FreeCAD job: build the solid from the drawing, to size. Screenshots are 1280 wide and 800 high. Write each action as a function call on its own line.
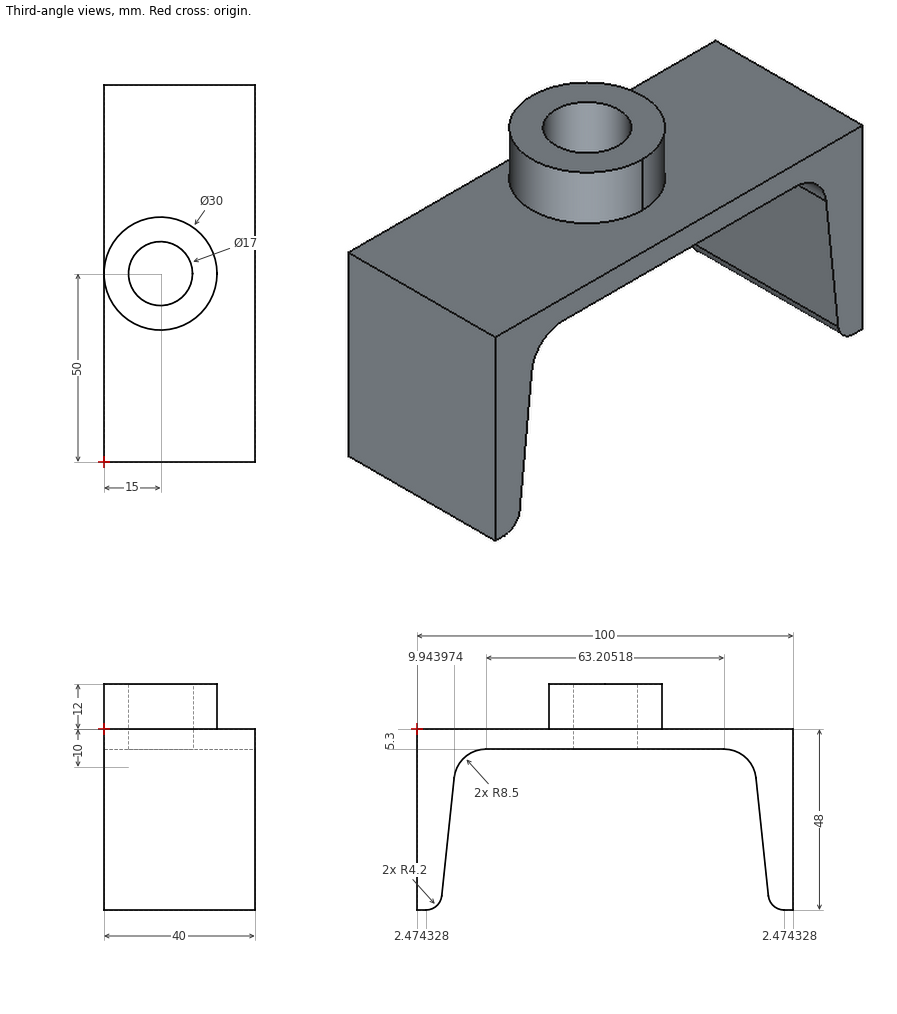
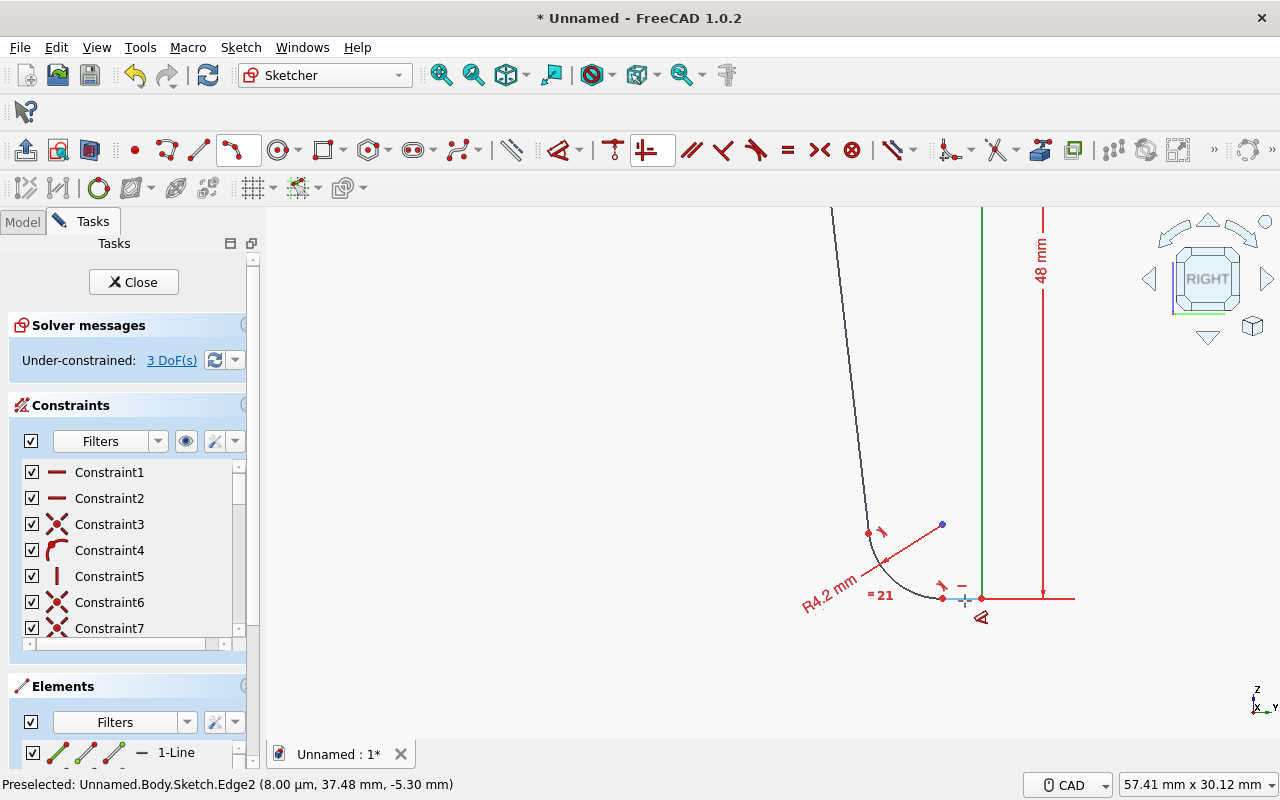
click(962, 599)
click(962, 633)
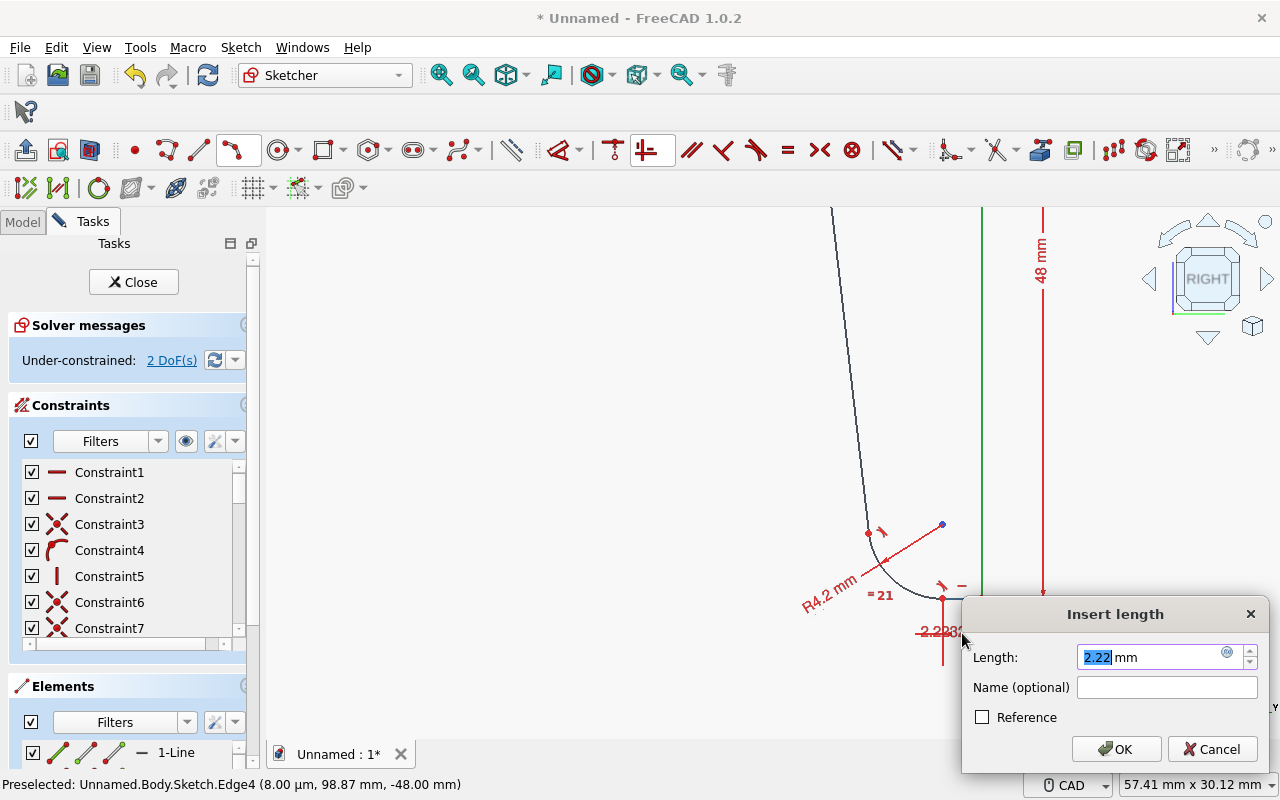
text(2.474328)
key(Return)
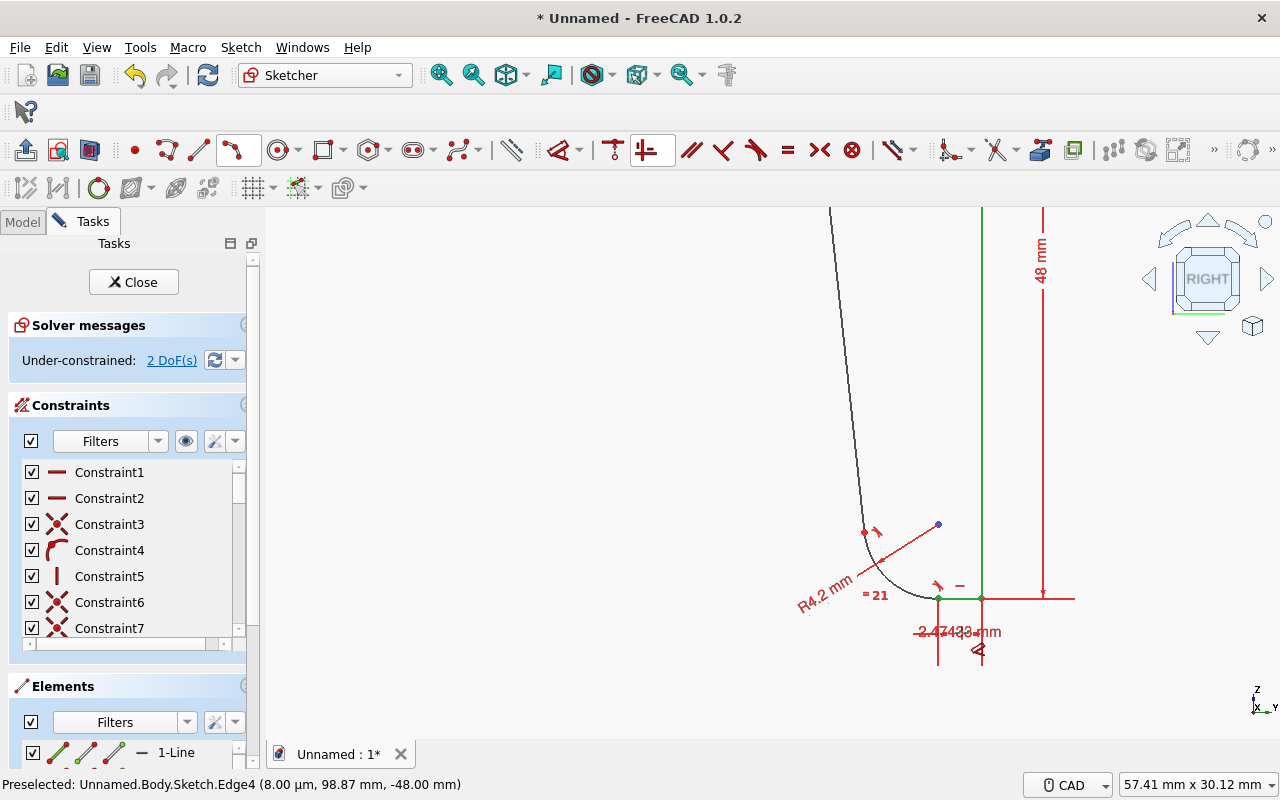
scroll(966, 601, down, 6)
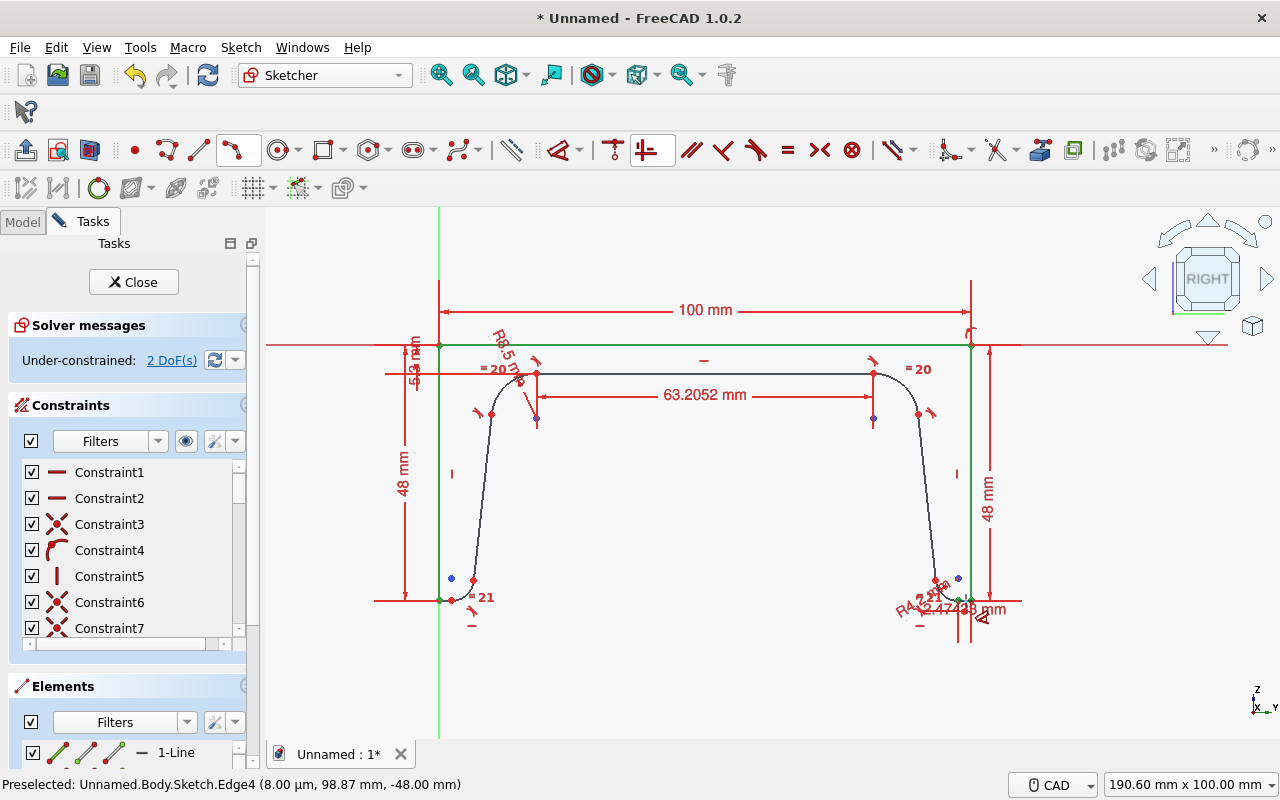
scroll(443, 601, up, 7)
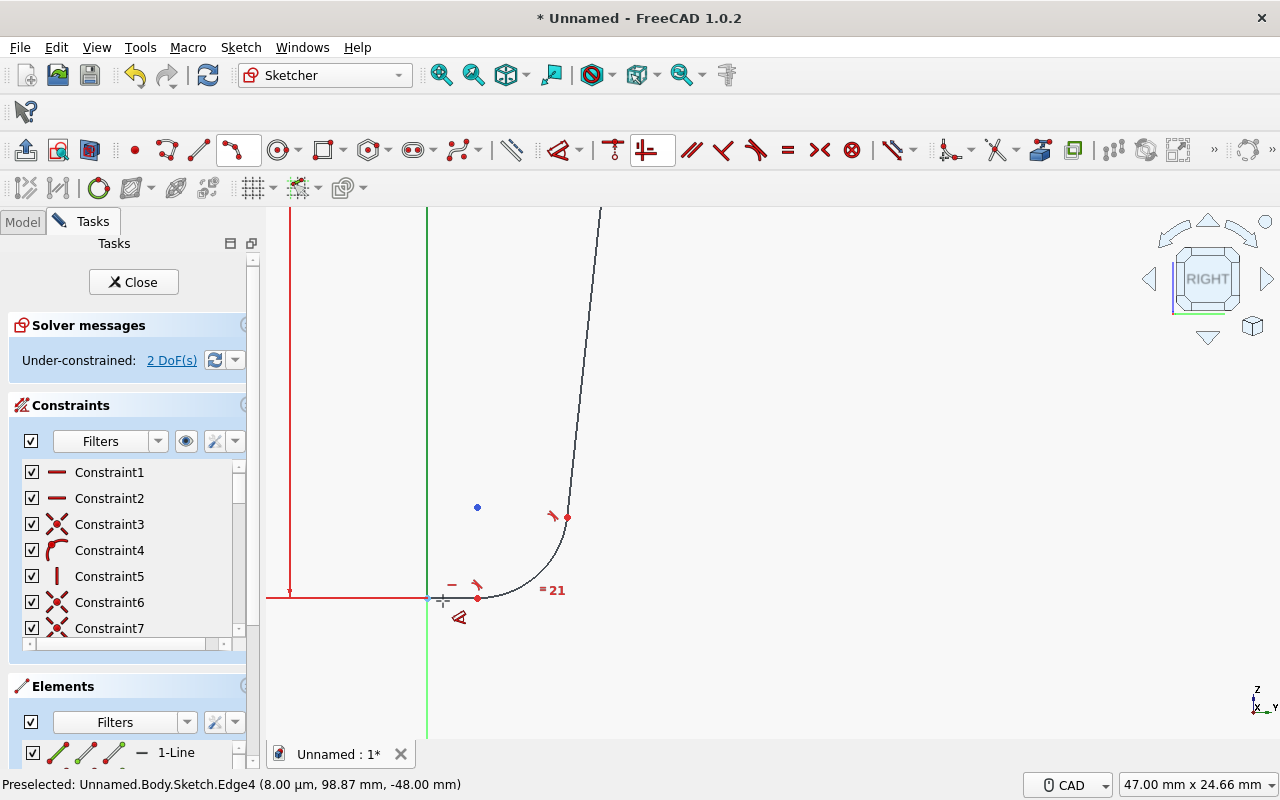
click(442, 598)
click(452, 632)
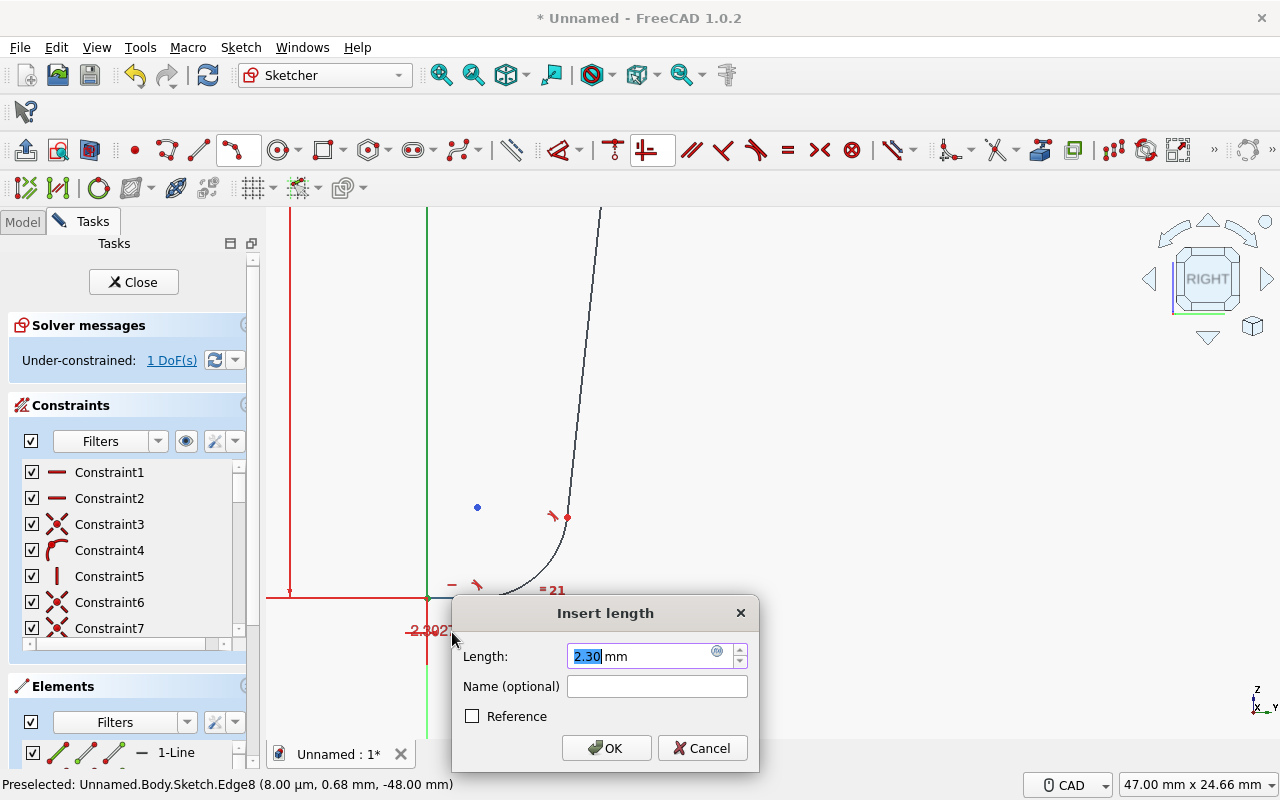
text(2.474328)
key(Return)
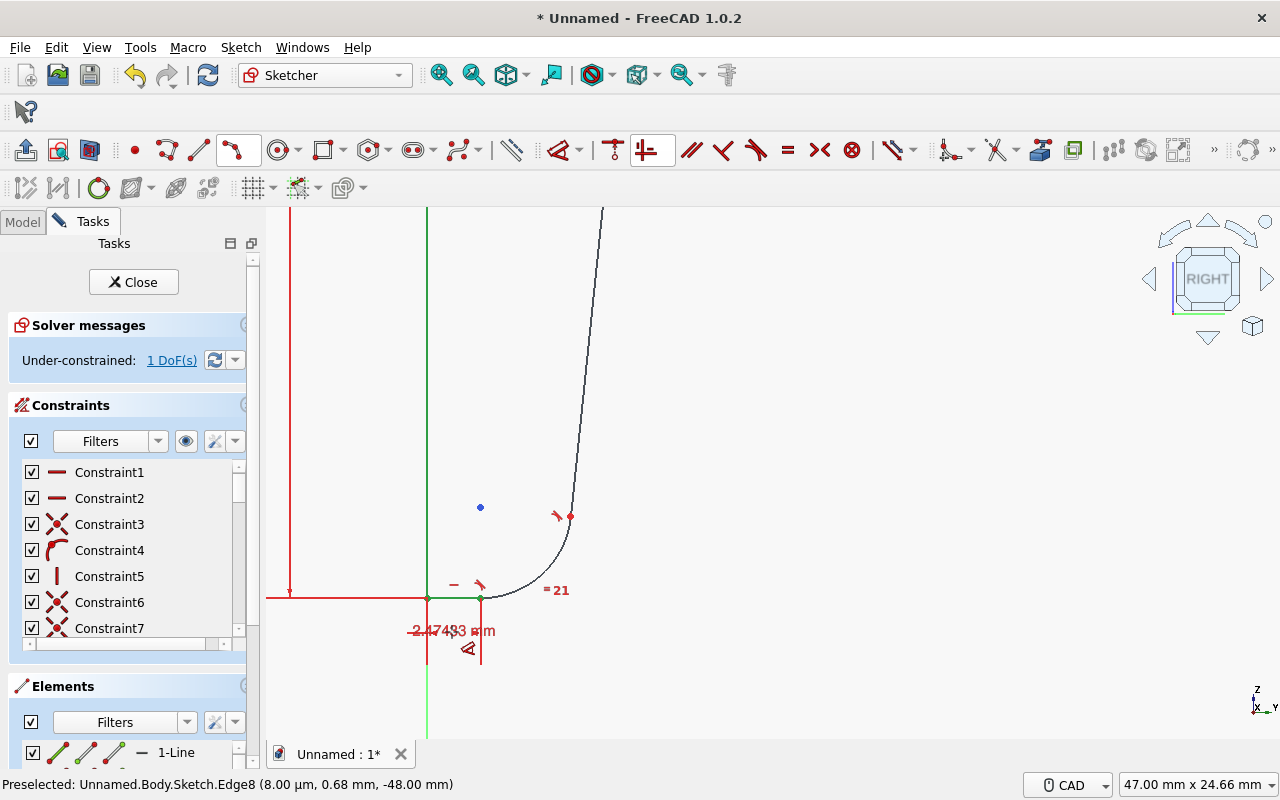
scroll(442, 602, down, 7)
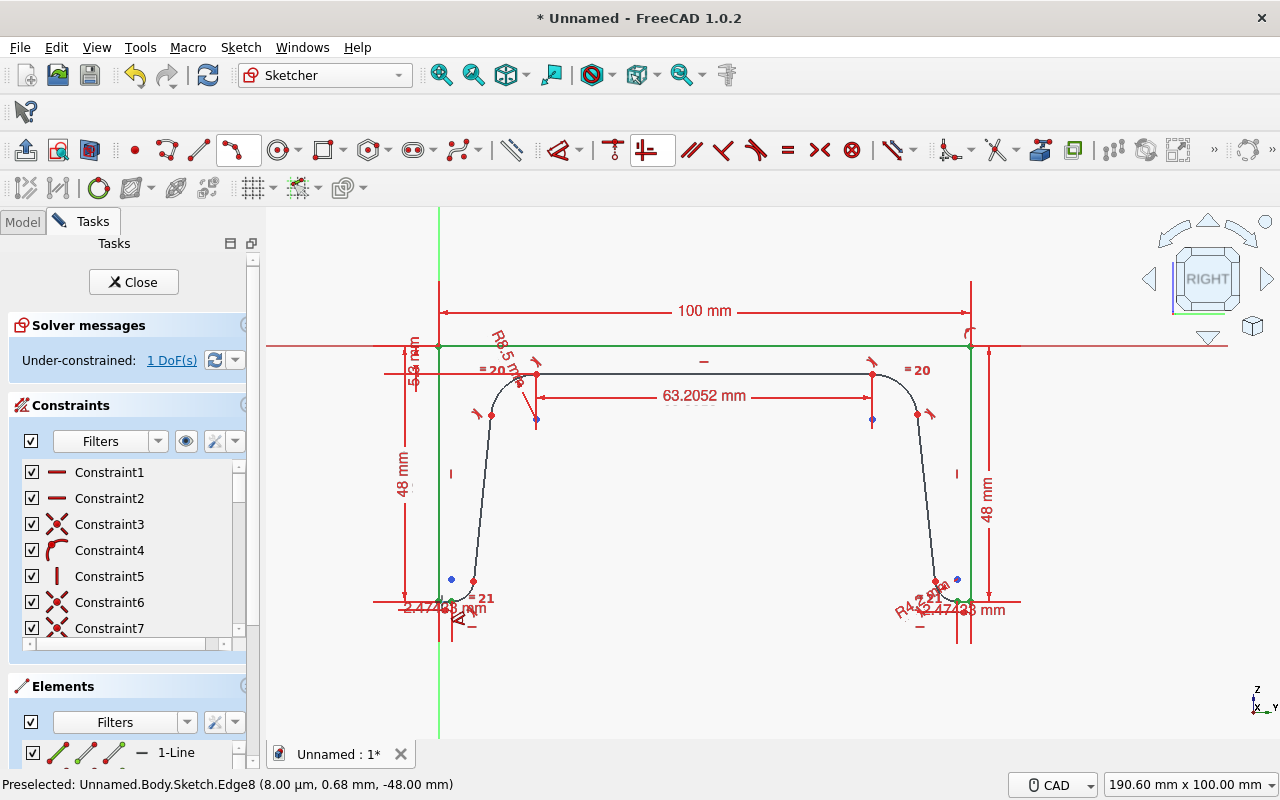
click(491, 415)
click(465, 312)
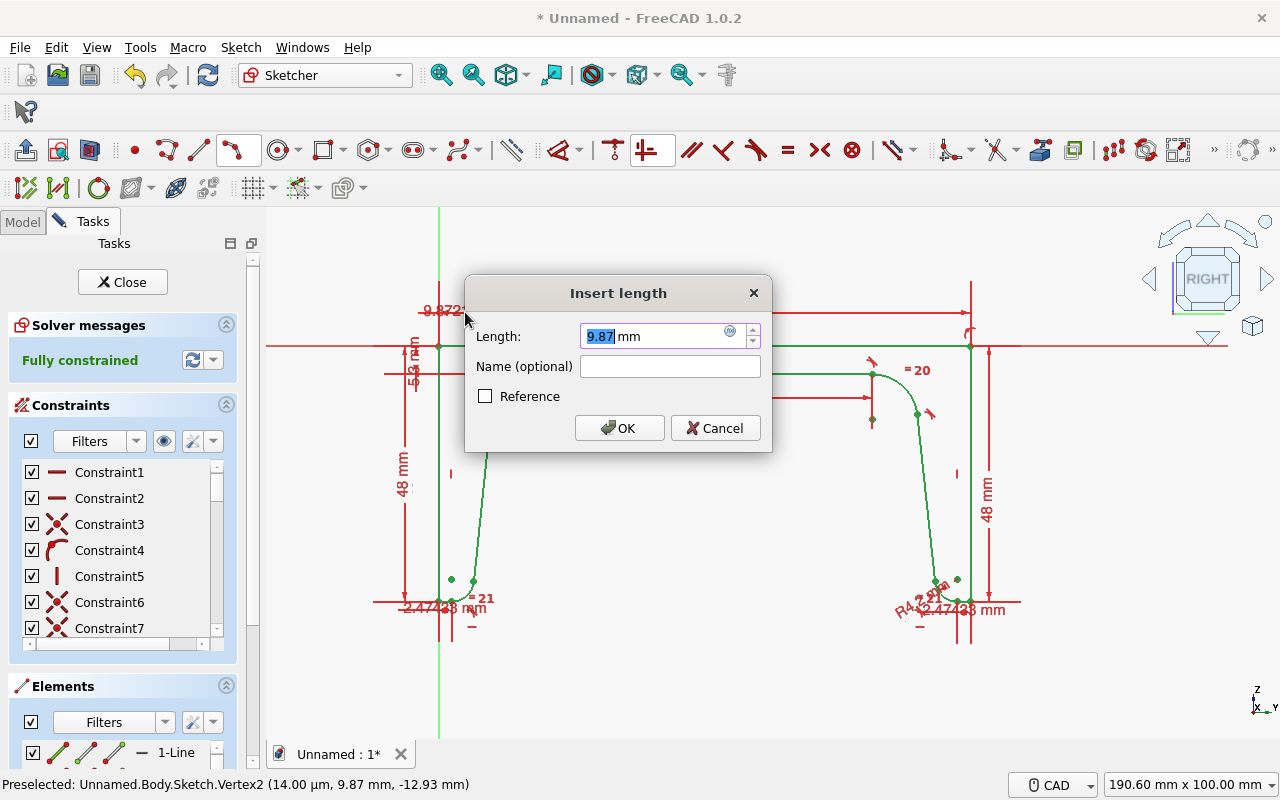
text(9.943974)
key(Return)
key(Escape)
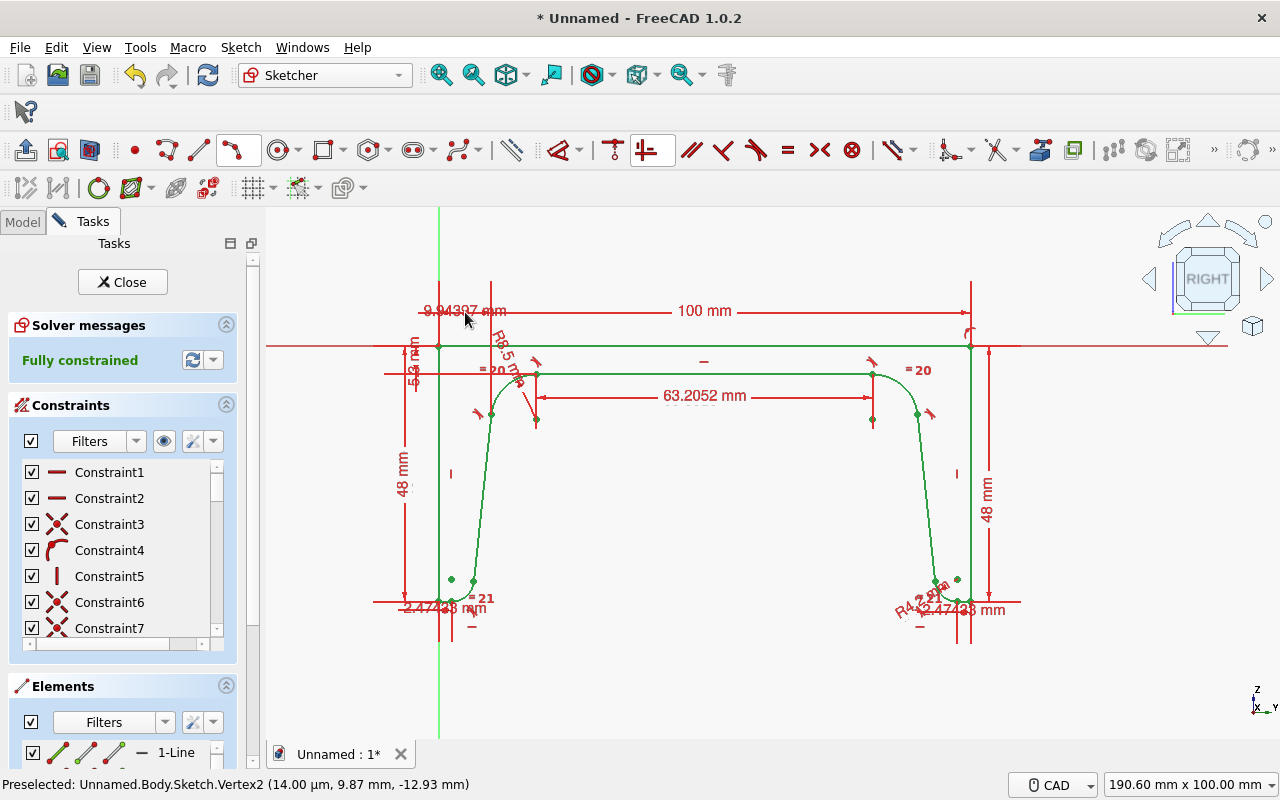
click(123, 282)